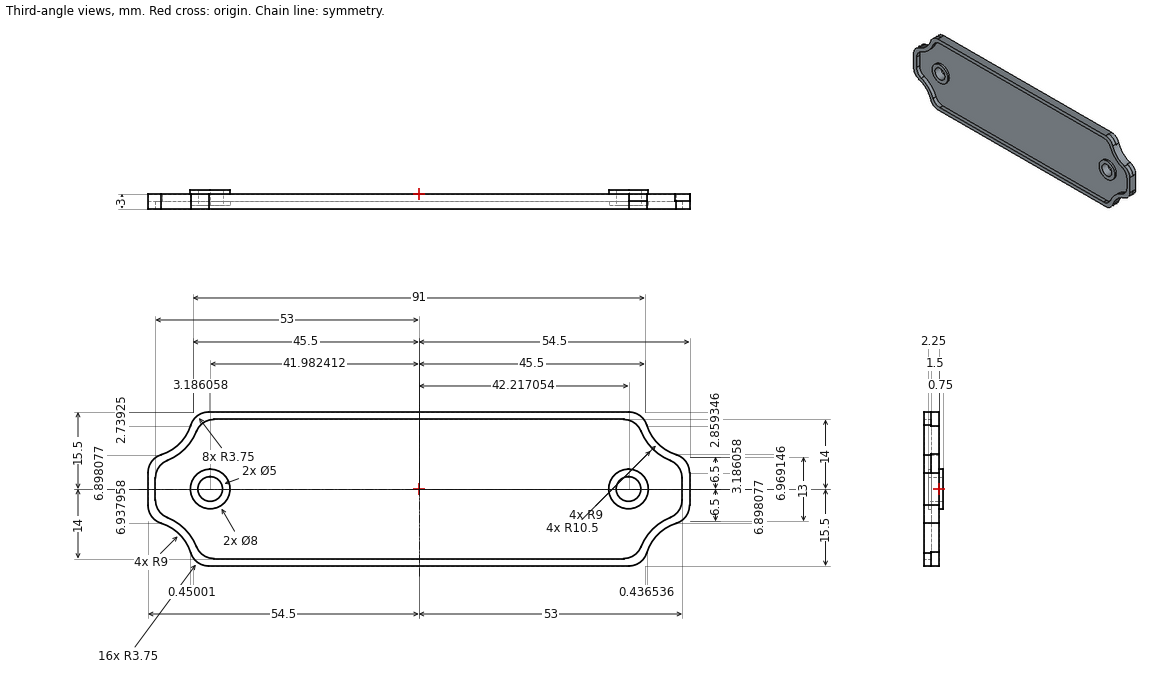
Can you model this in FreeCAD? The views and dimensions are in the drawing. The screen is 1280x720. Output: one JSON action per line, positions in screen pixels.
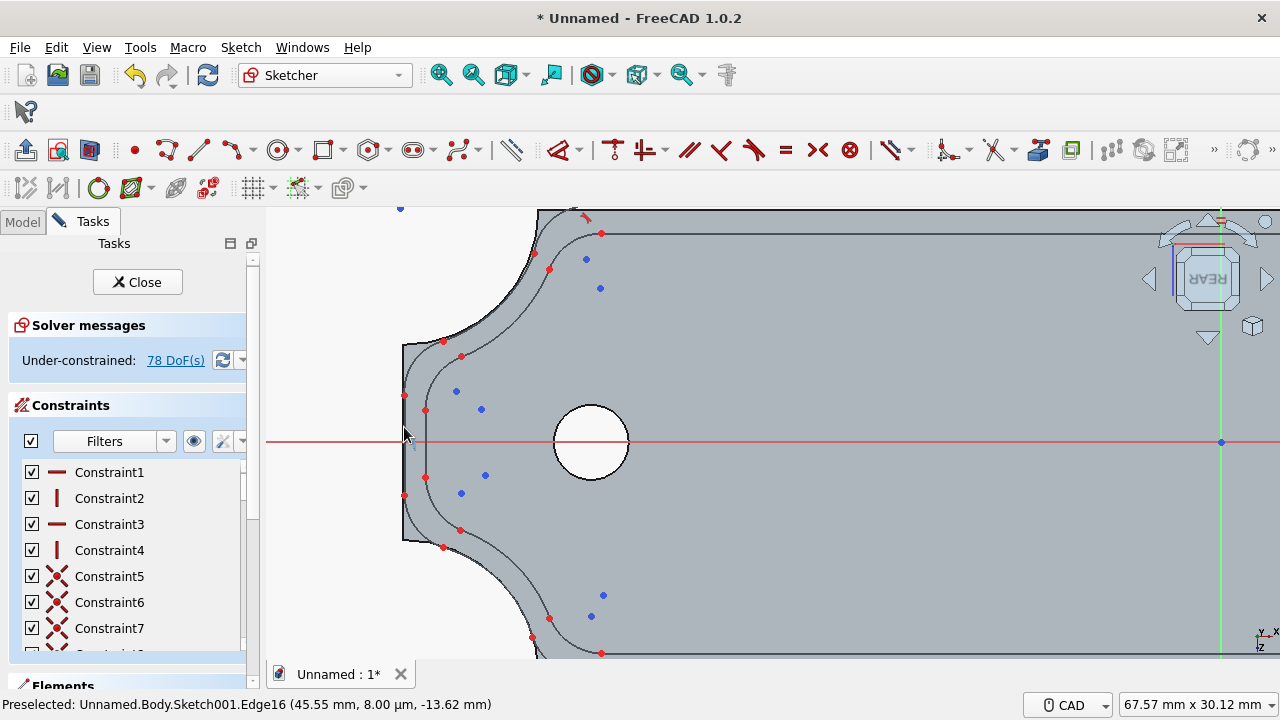
{"action": "left_click", "coordinate": [405, 426]}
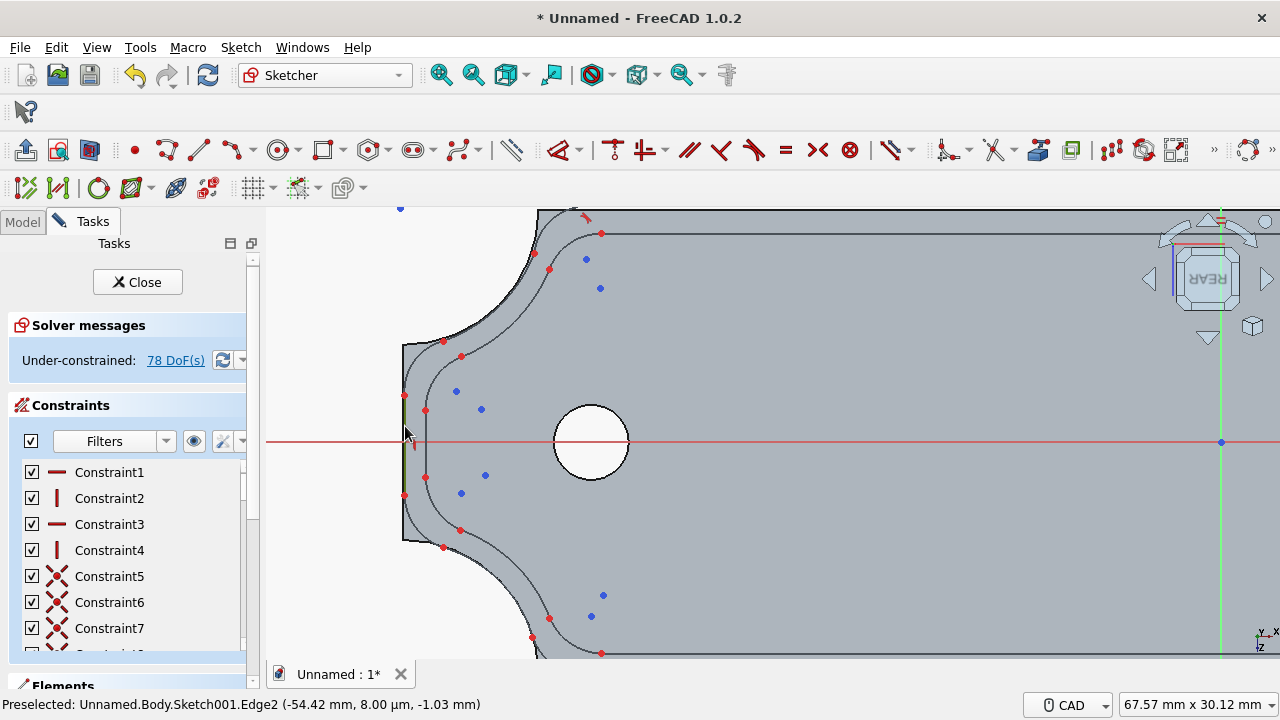
{"action": "left_click", "coordinate": [424, 351]}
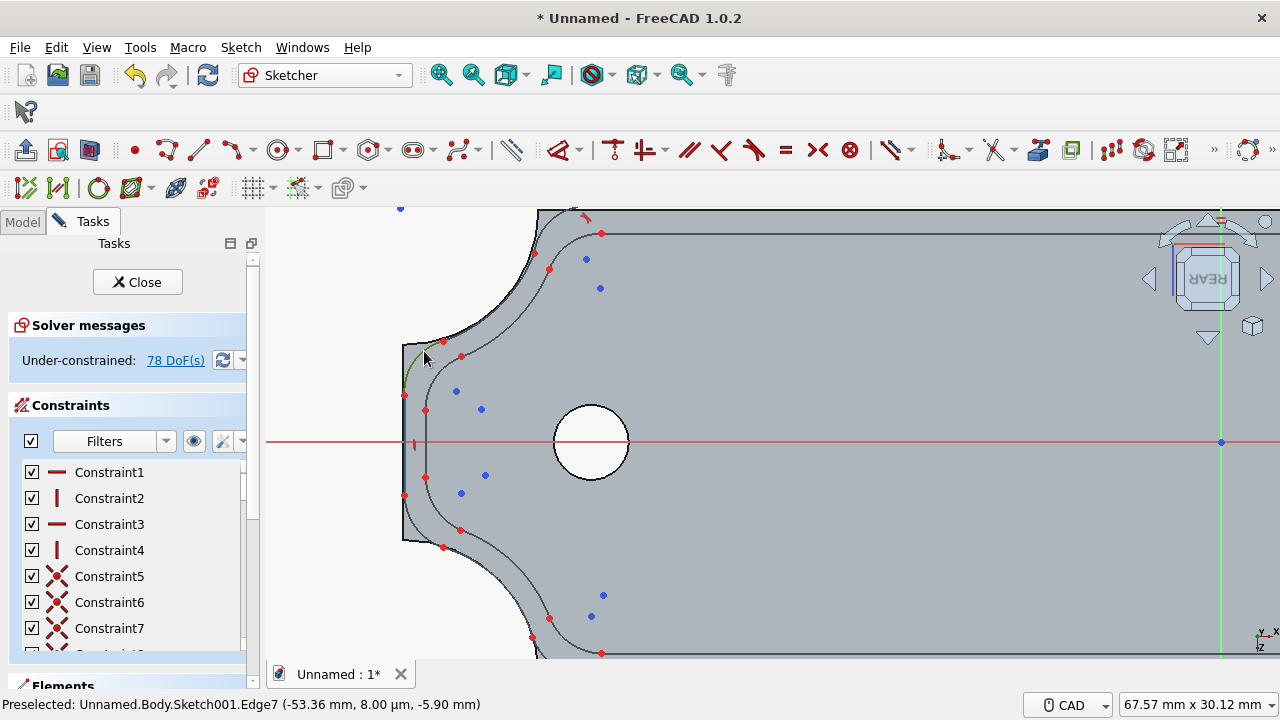
{"action": "left_click", "coordinate": [754, 150]}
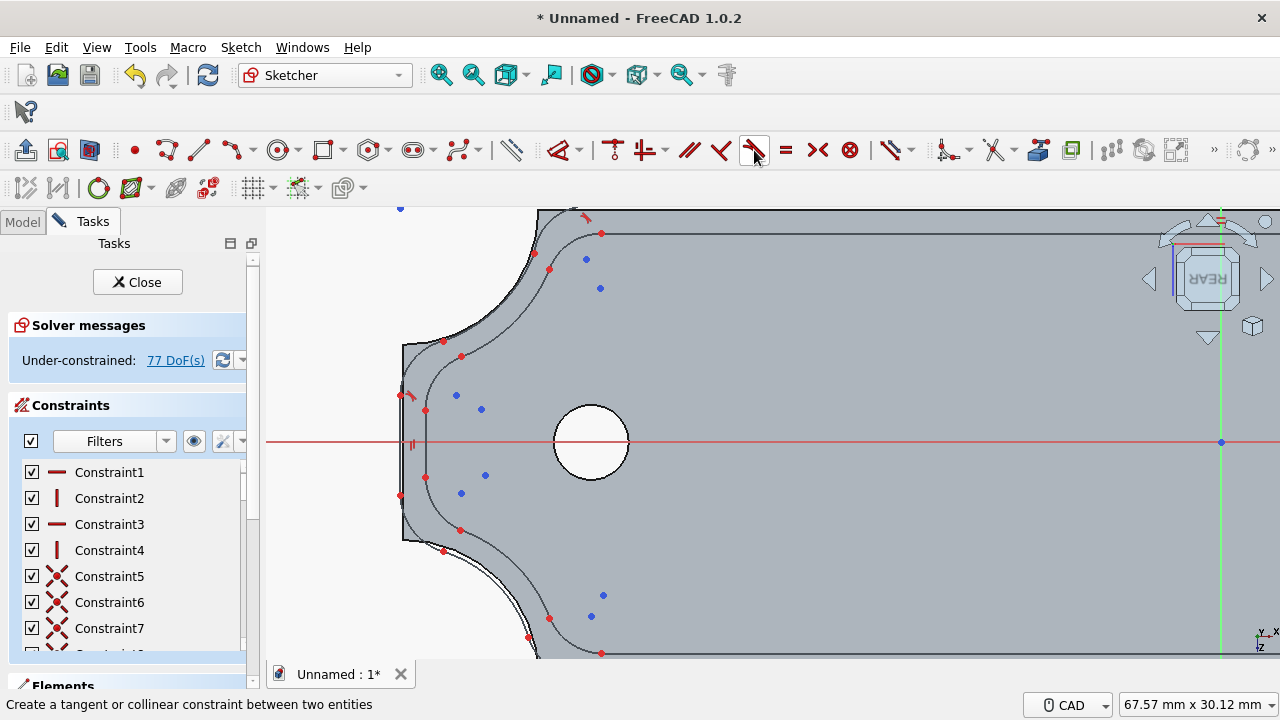
{"action": "left_click", "coordinate": [400, 426]}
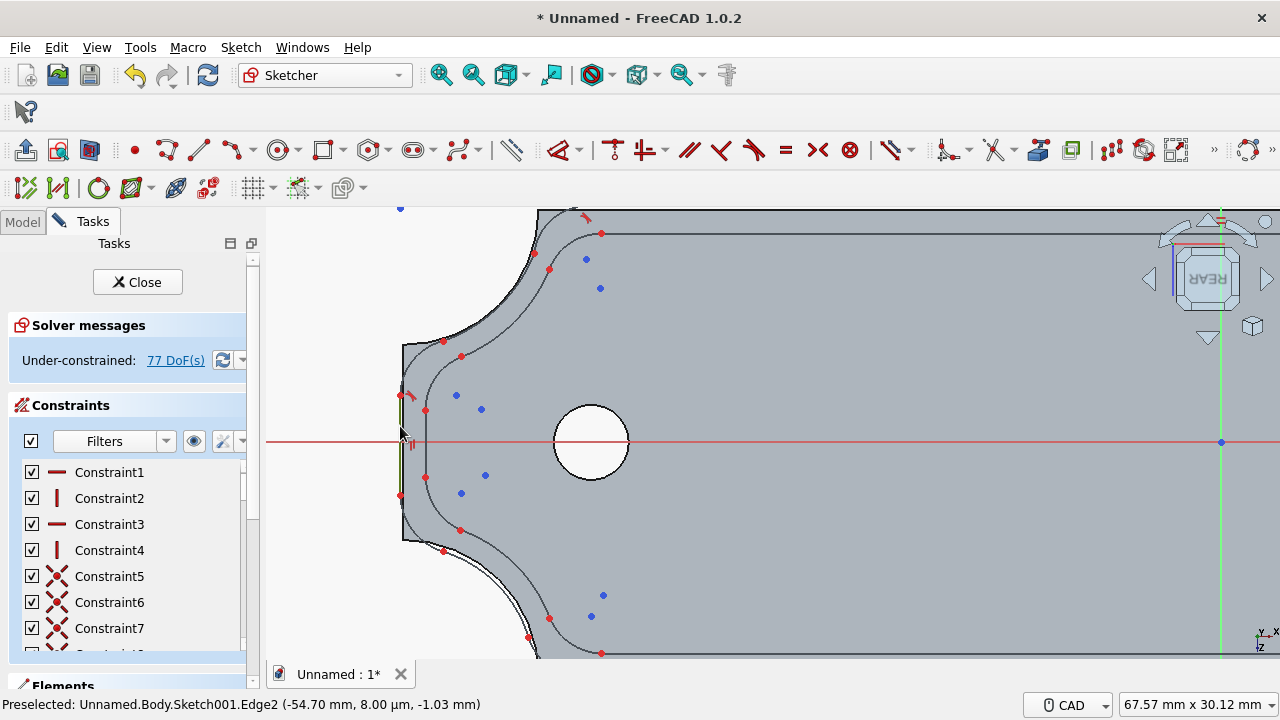
{"action": "left_click", "coordinate": [405, 517]}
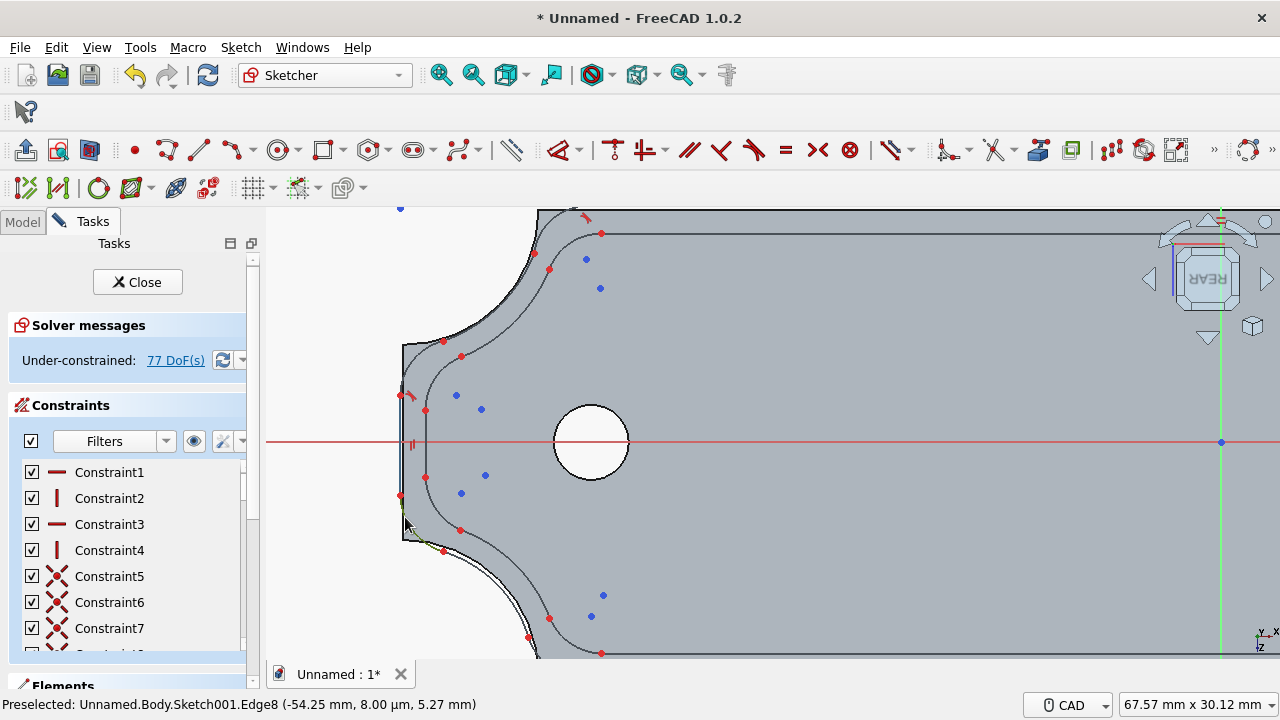
{"action": "left_click", "coordinate": [754, 150]}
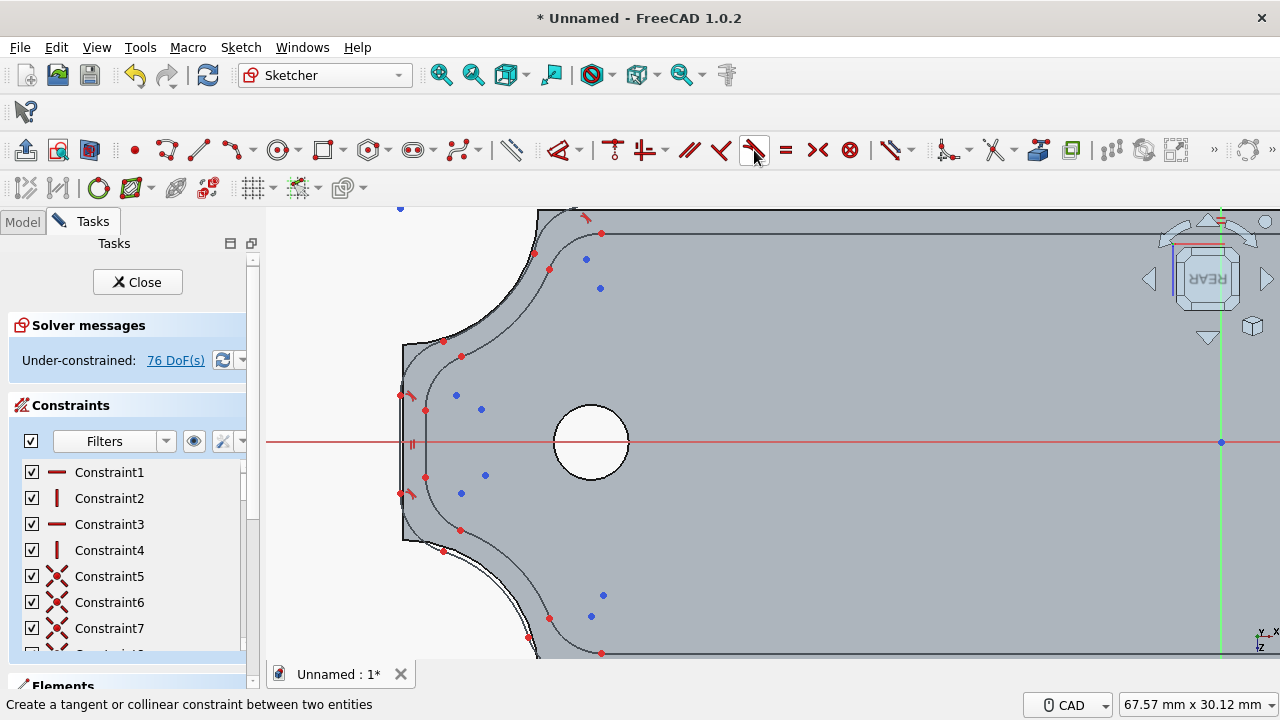
{"action": "scroll", "coordinate": [404, 428], "scroll_direction": "down", "scroll_amount": 5}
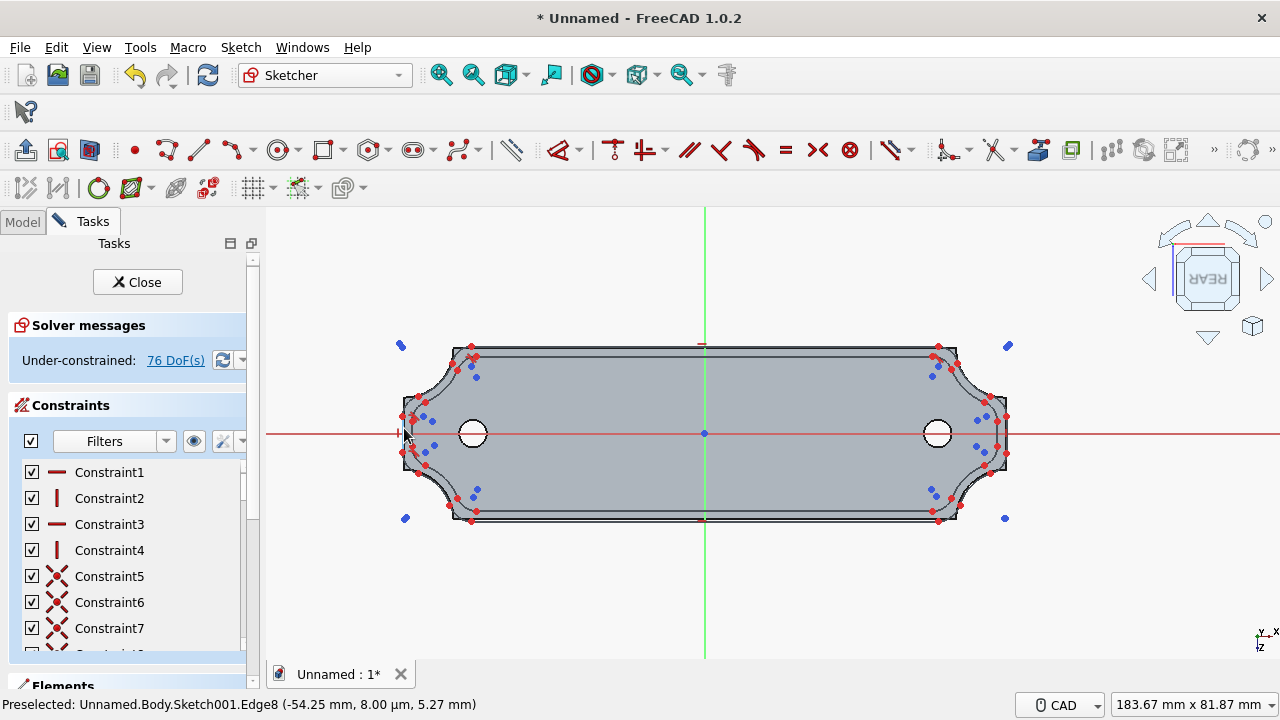
{"action": "scroll", "coordinate": [611, 522], "scroll_direction": "up", "scroll_amount": 2}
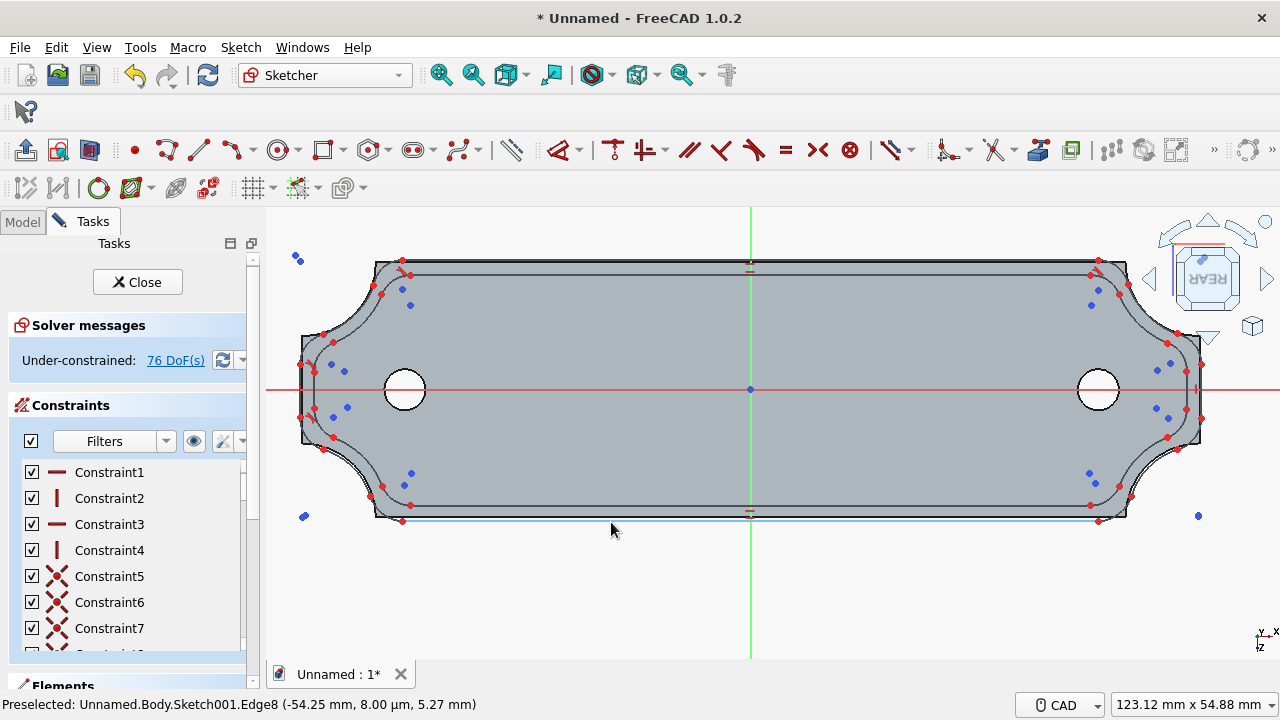
{"action": "left_click", "coordinate": [611, 521]}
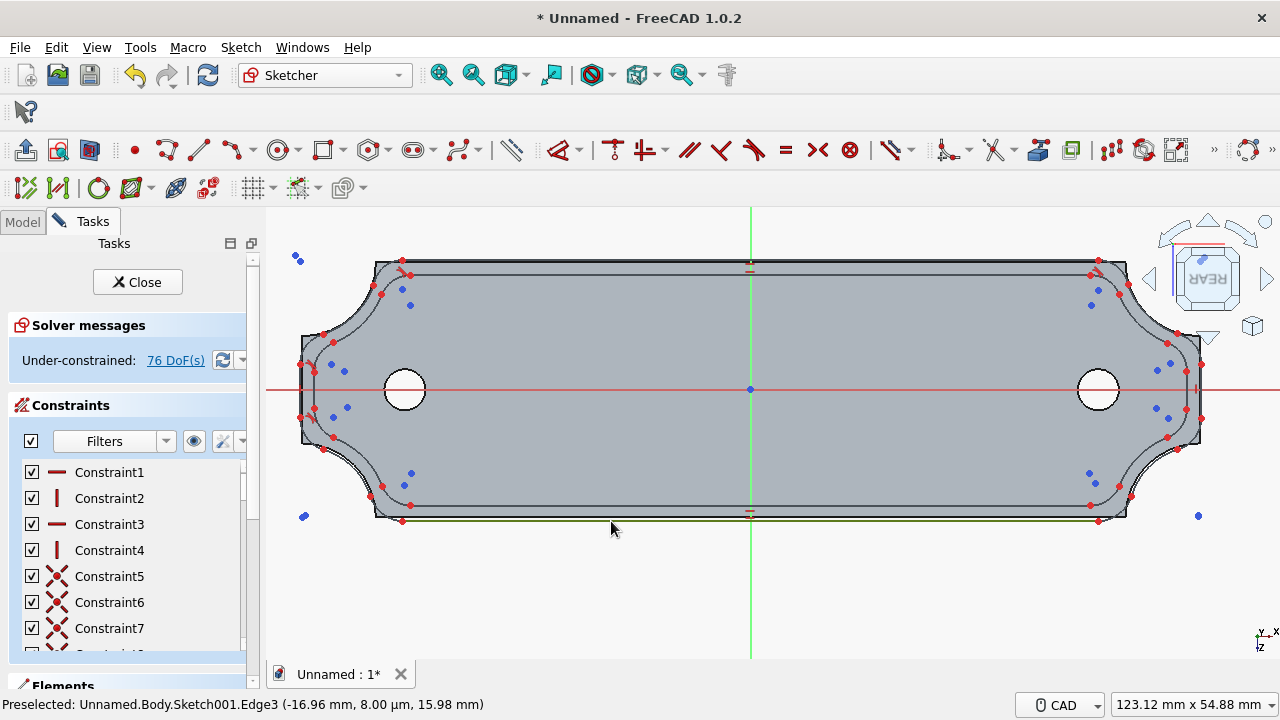
{"action": "left_click", "coordinate": [377, 508]}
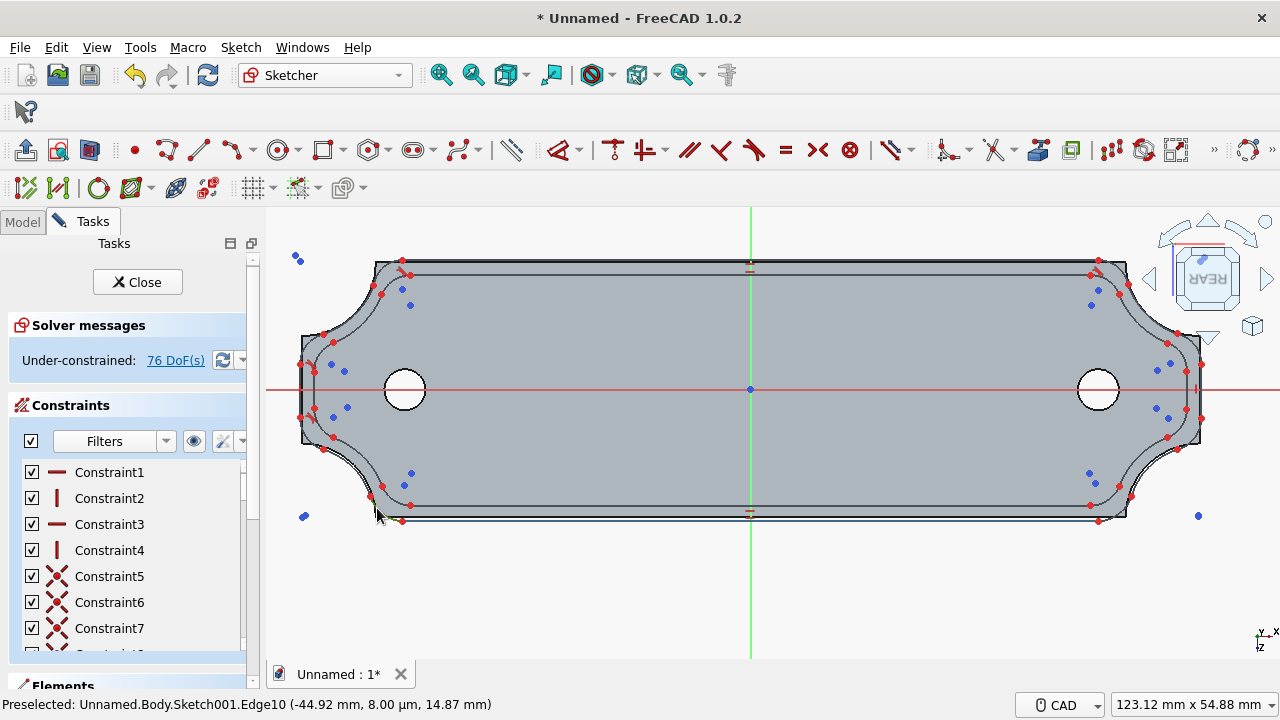
{"action": "left_click", "coordinate": [754, 150]}